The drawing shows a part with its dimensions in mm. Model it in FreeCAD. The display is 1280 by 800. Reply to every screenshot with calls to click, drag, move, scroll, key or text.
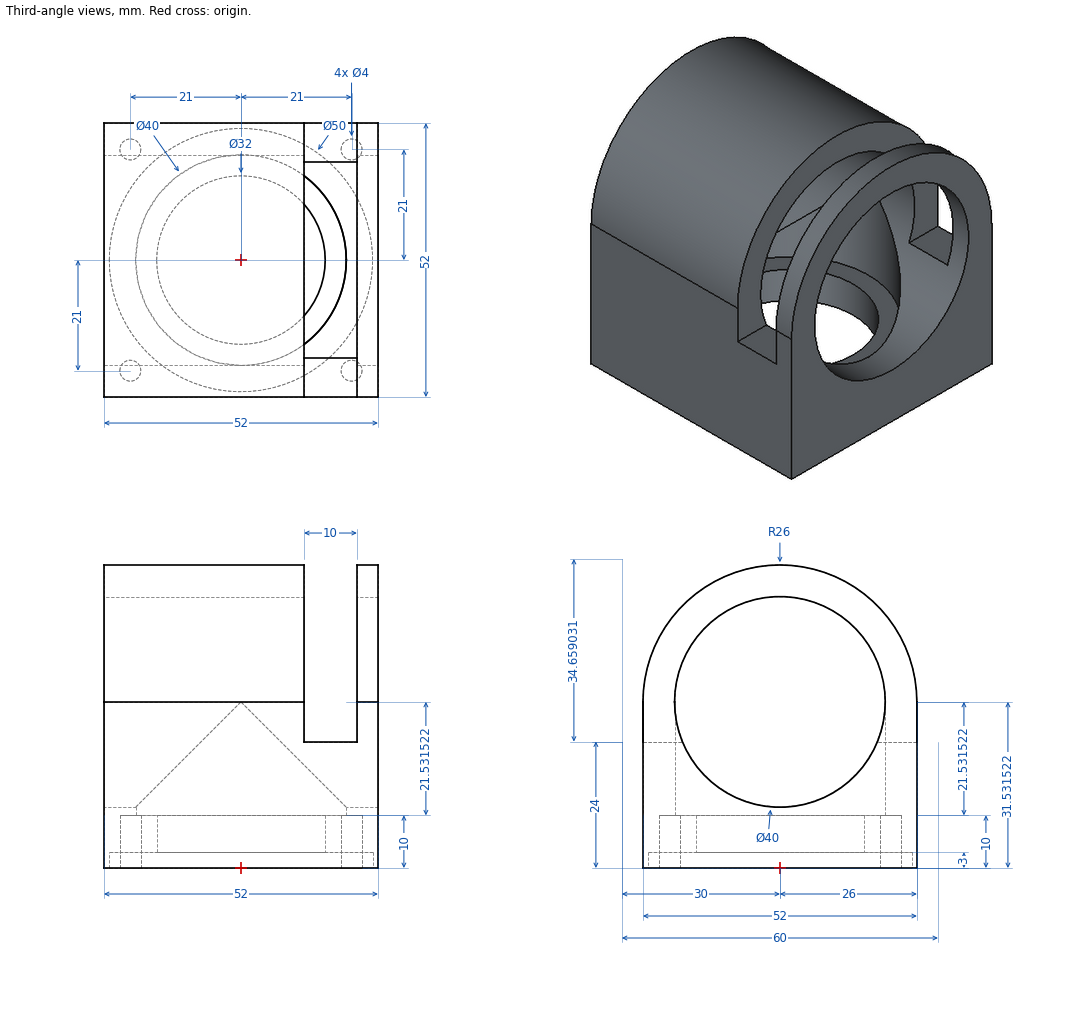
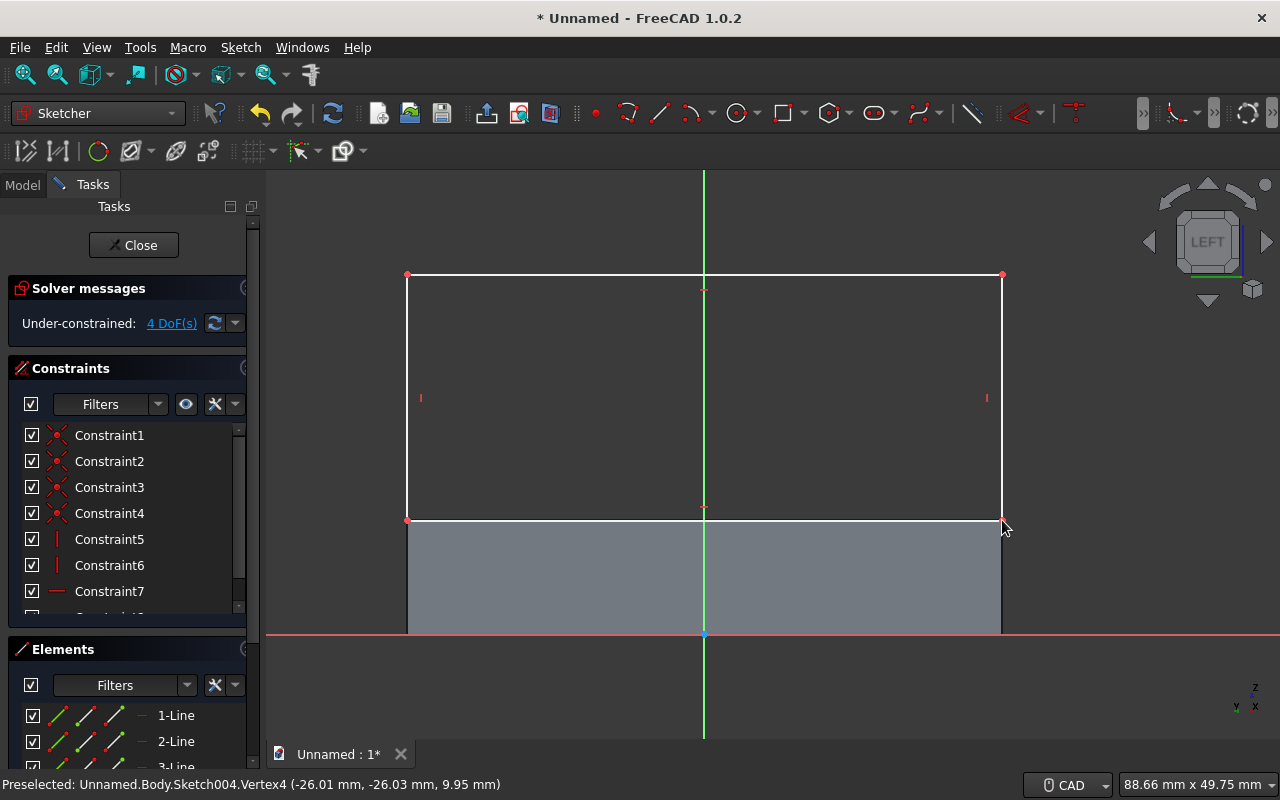
click(1020, 114)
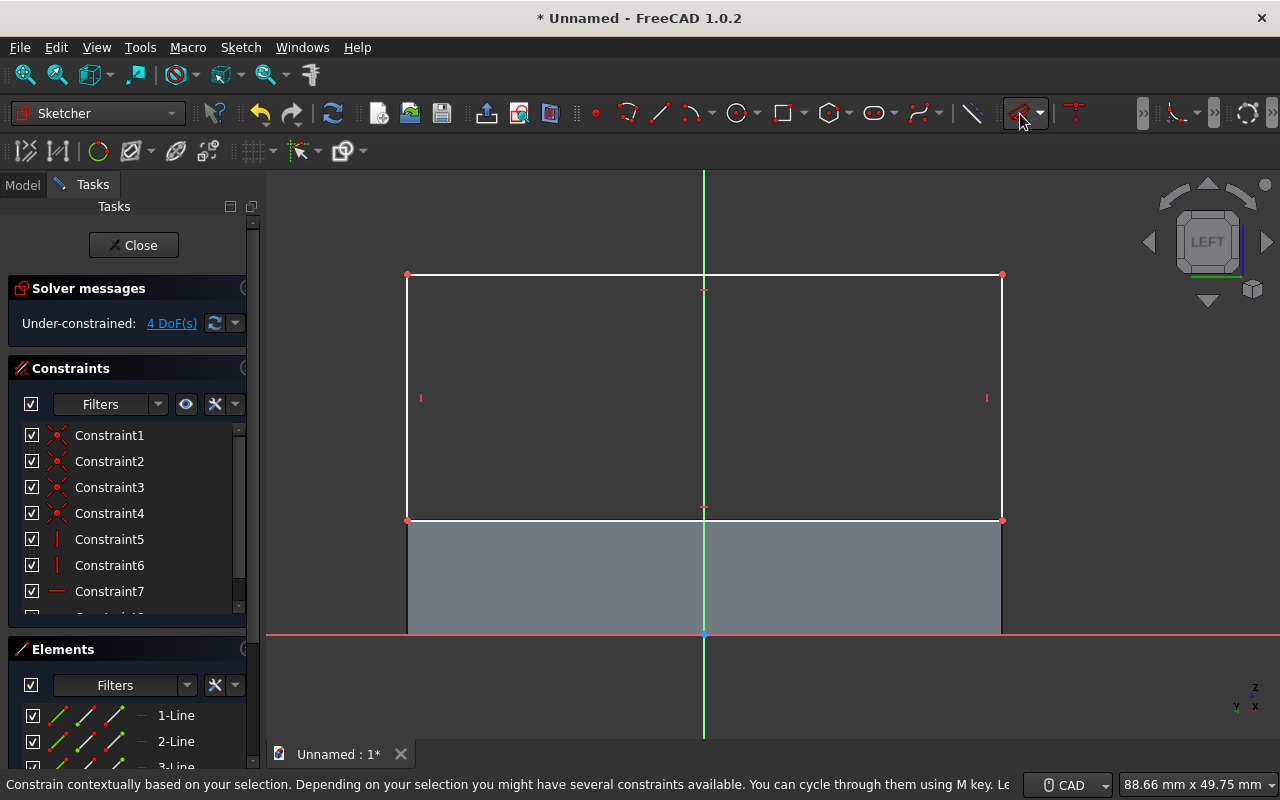
click(585, 521)
click(568, 555)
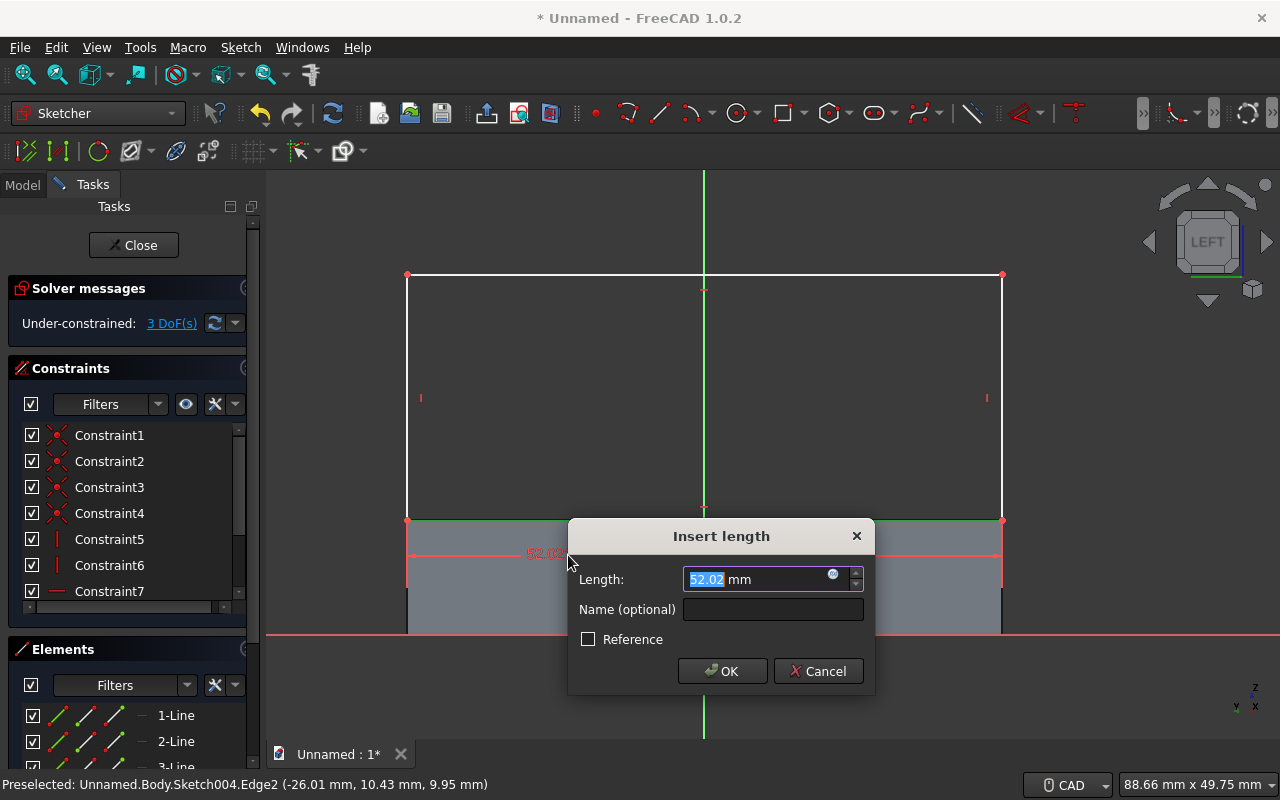
text(52)
key(Return)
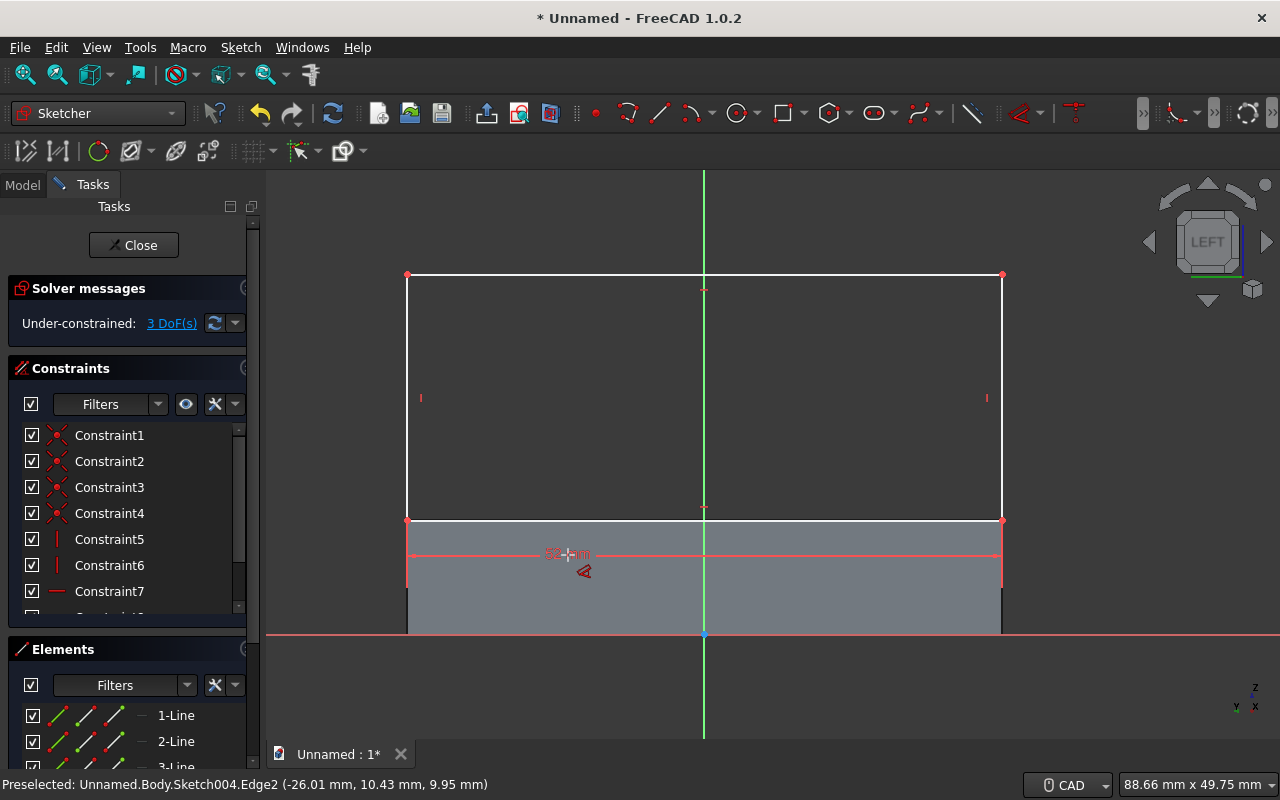
click(407, 275)
click(556, 669)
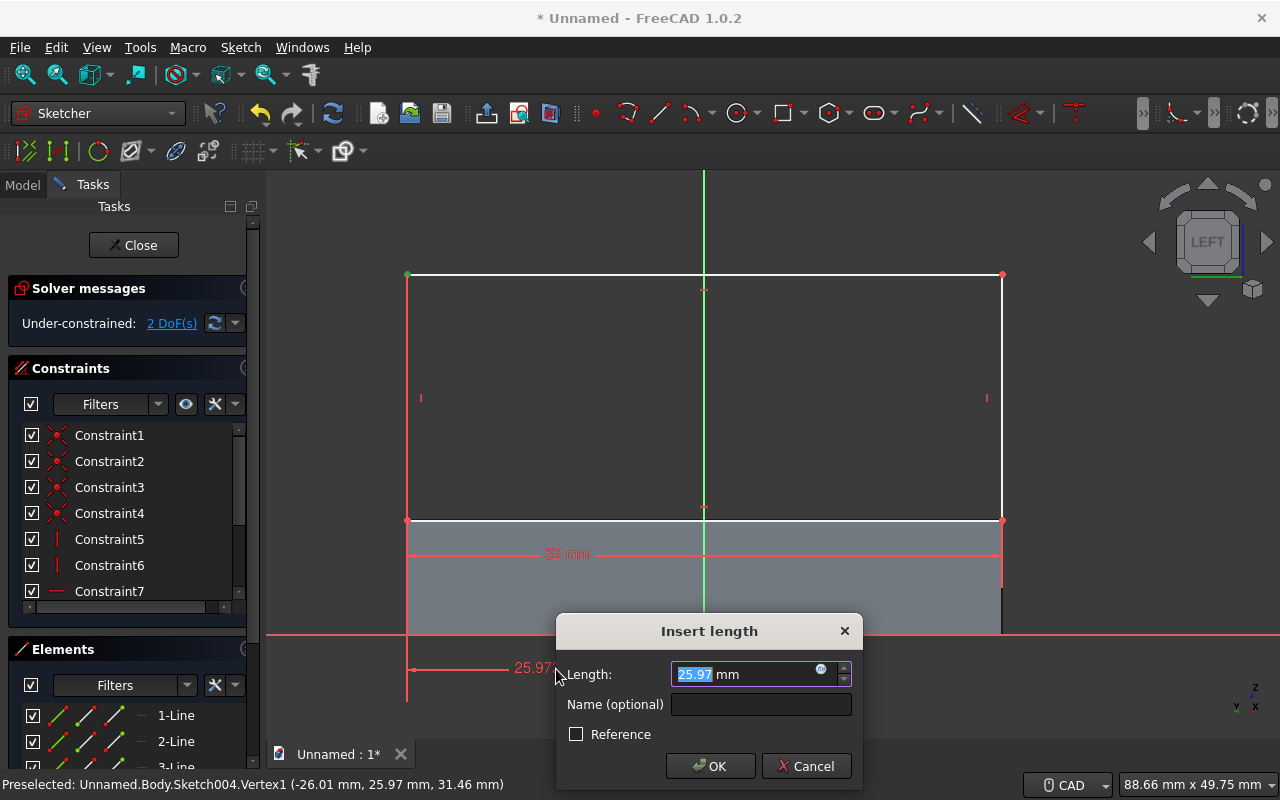
text(26)
key(Return)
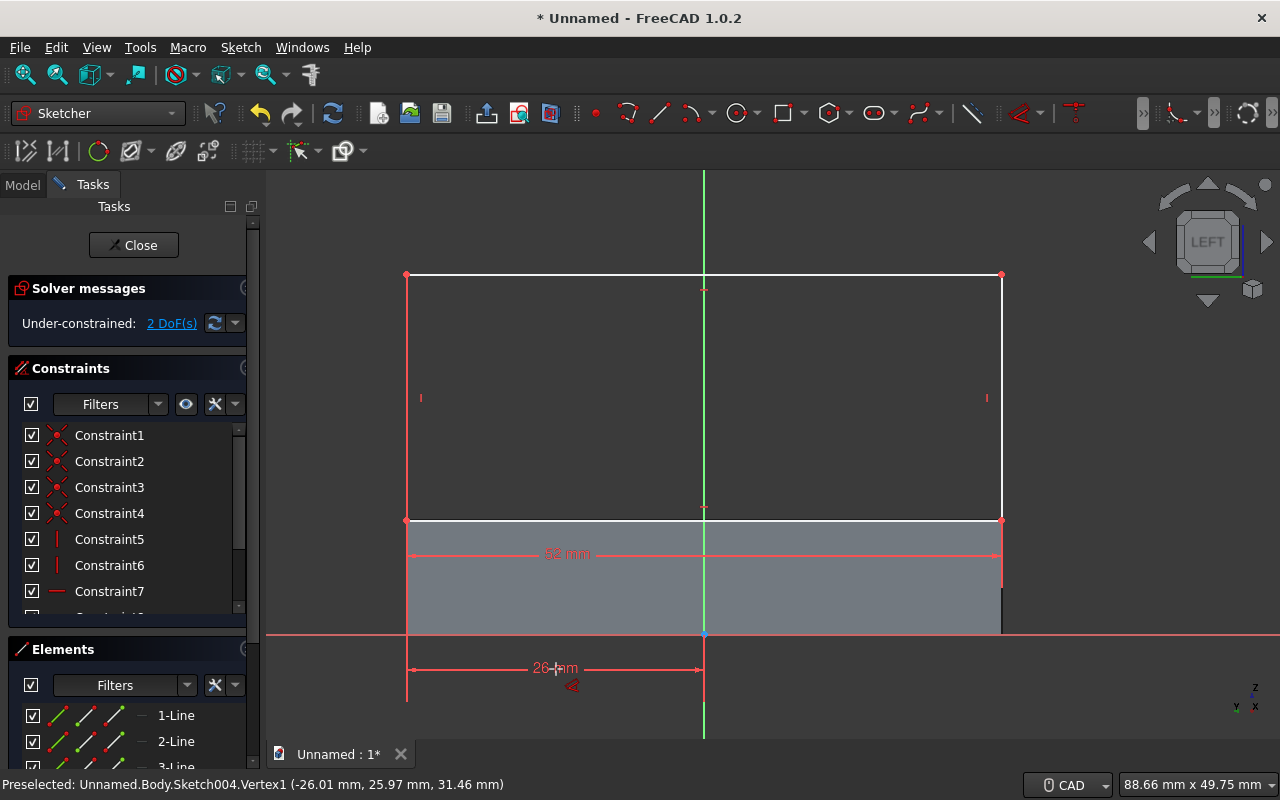
click(407, 521)
click(373, 578)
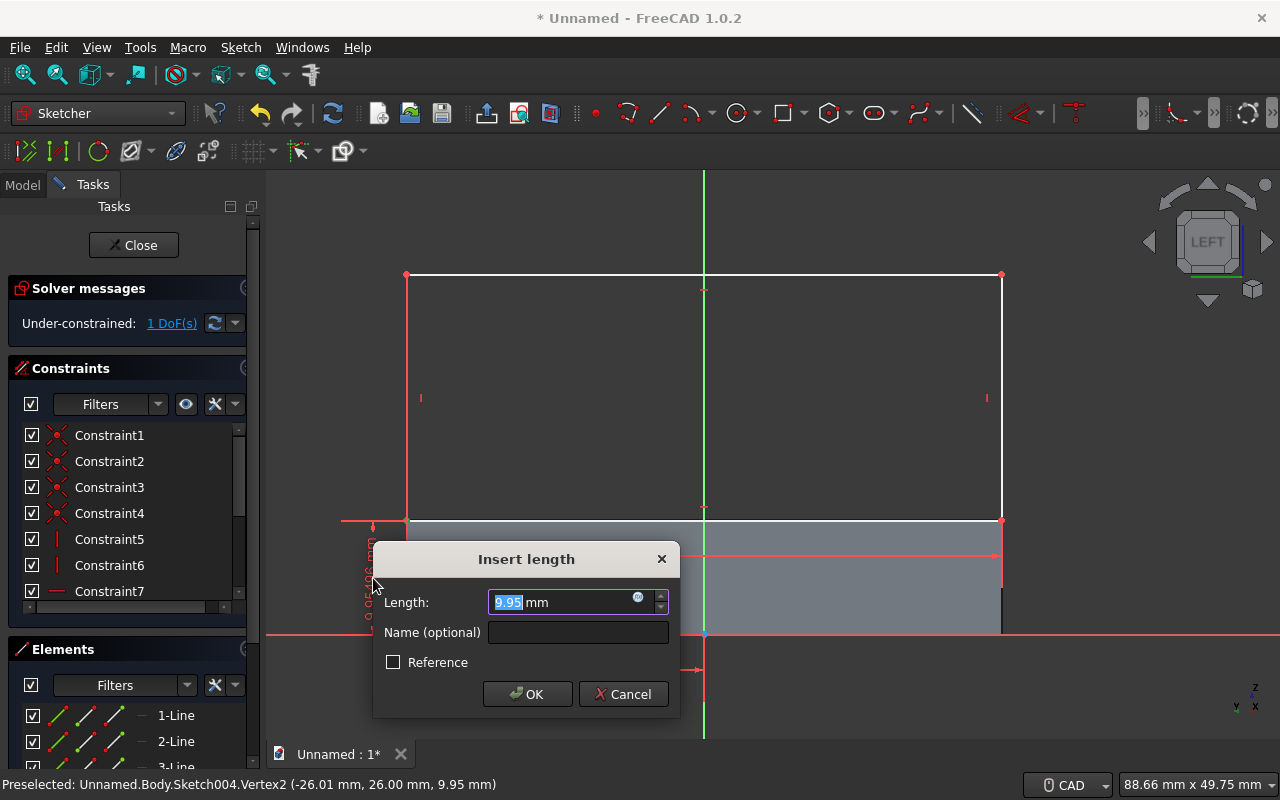
text(10)
key(Return)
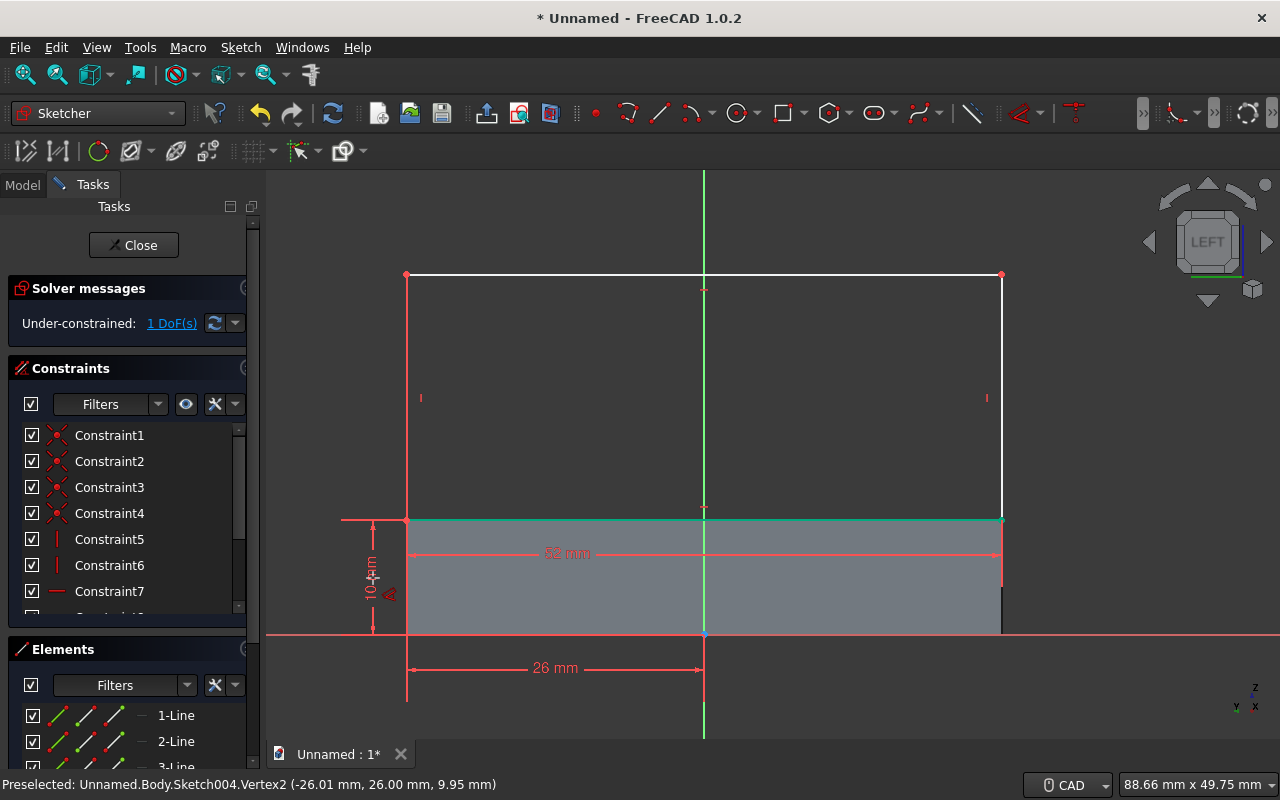
click(407, 349)
click(373, 398)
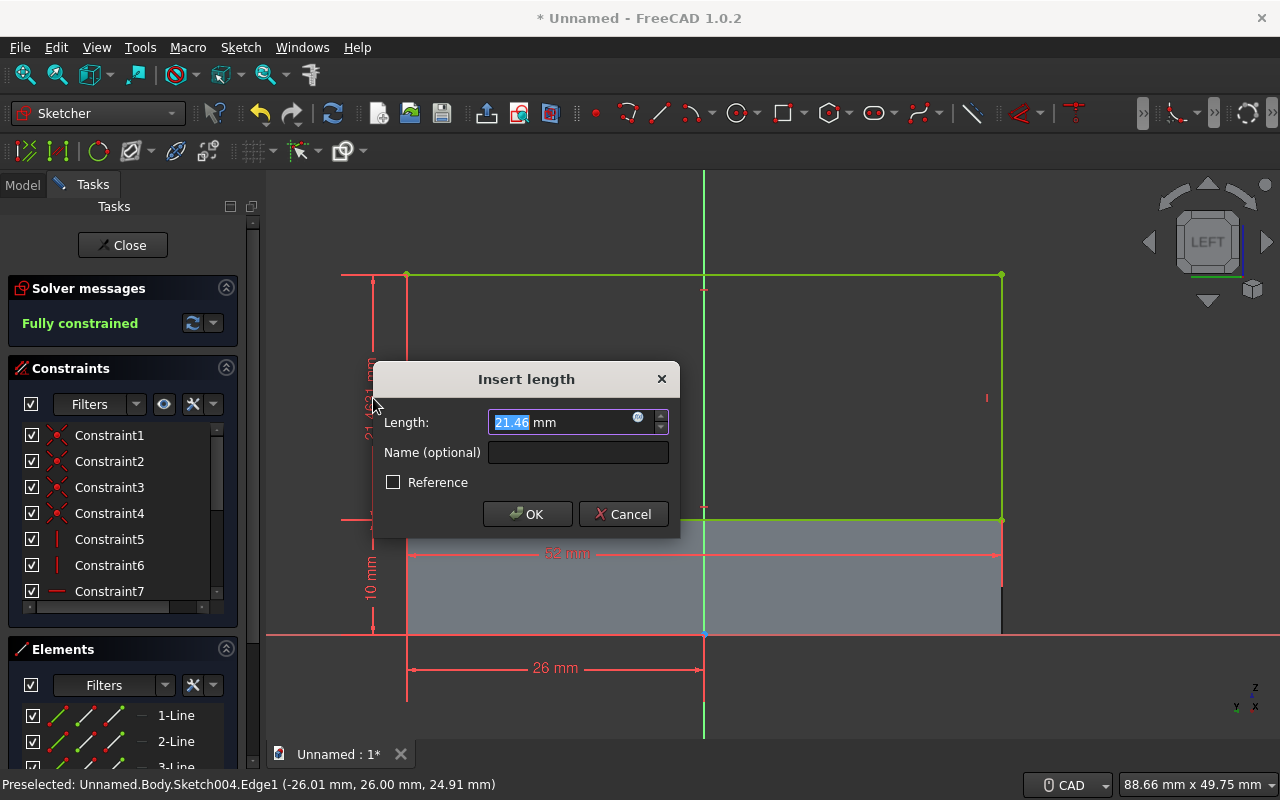
text(21.531522)
key(Return)
key(Escape)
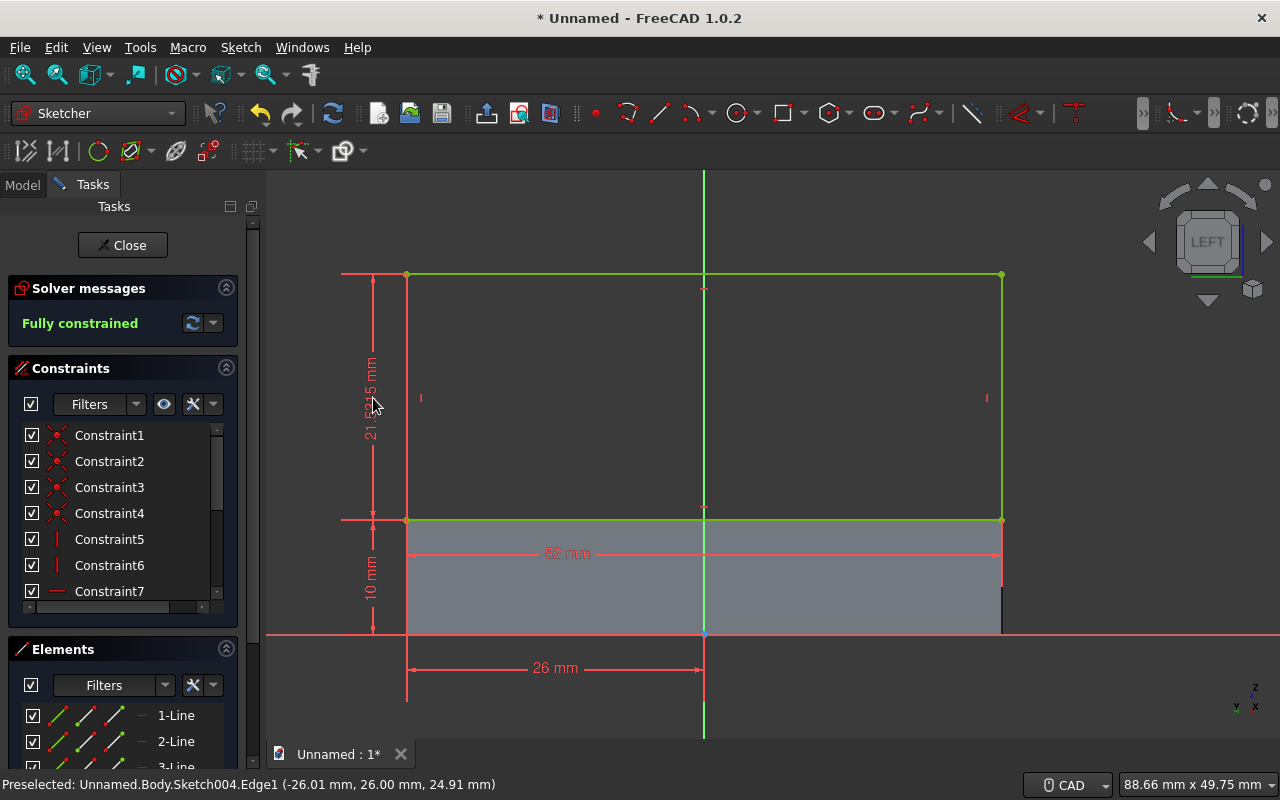
click(123, 245)